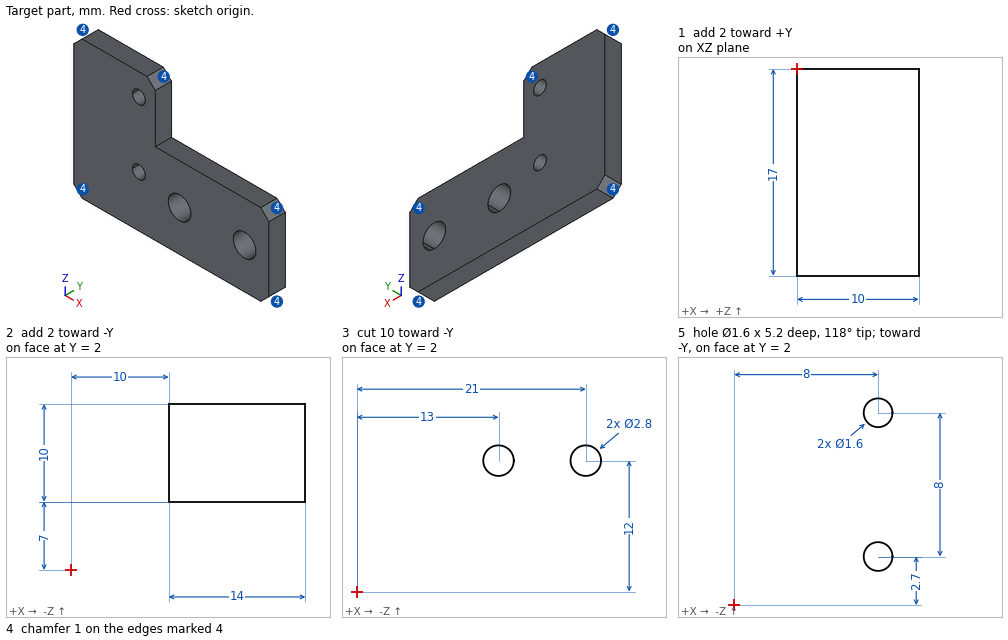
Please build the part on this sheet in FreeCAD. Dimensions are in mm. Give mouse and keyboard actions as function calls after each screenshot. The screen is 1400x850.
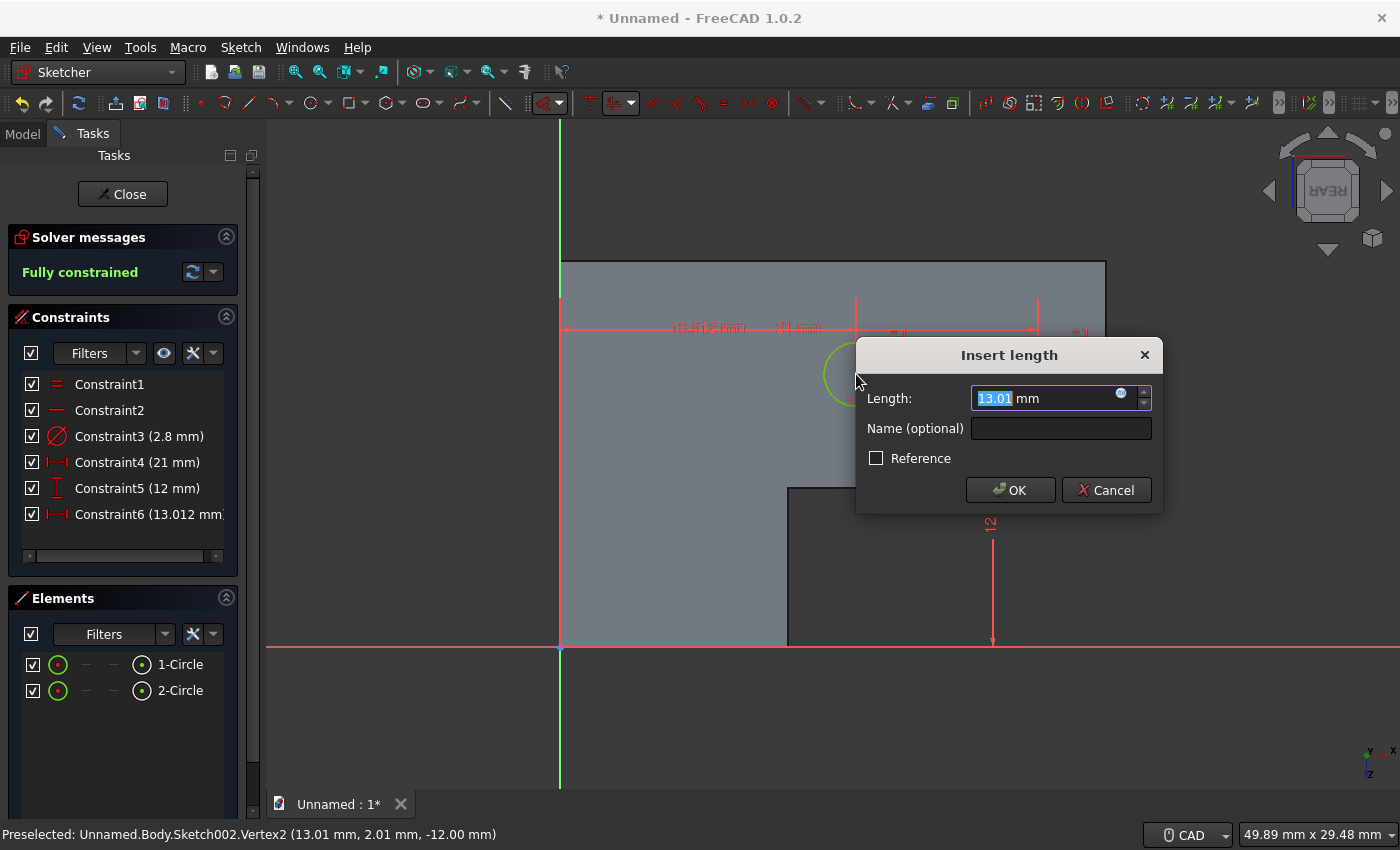
text(13)
key(Return)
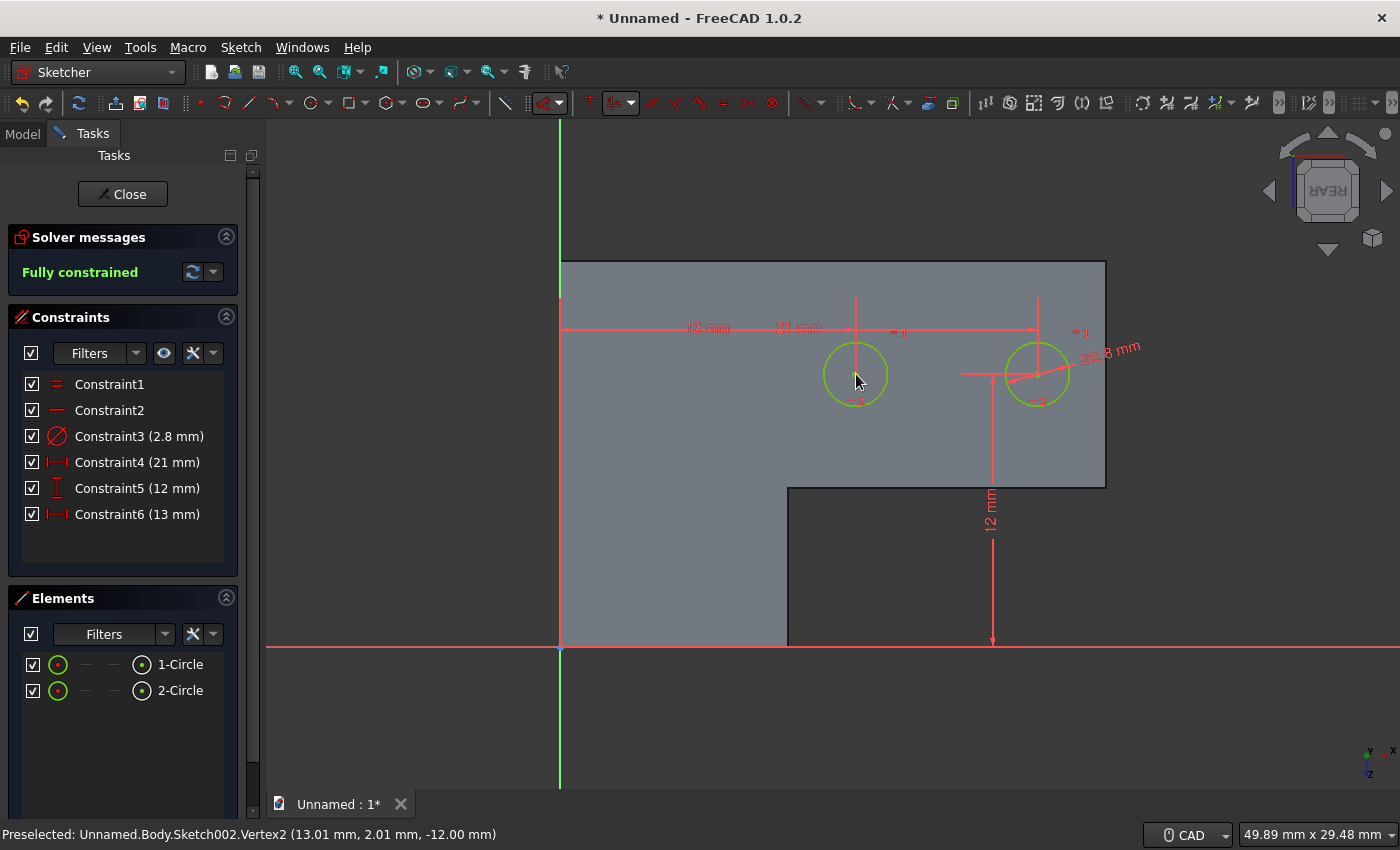
click(123, 194)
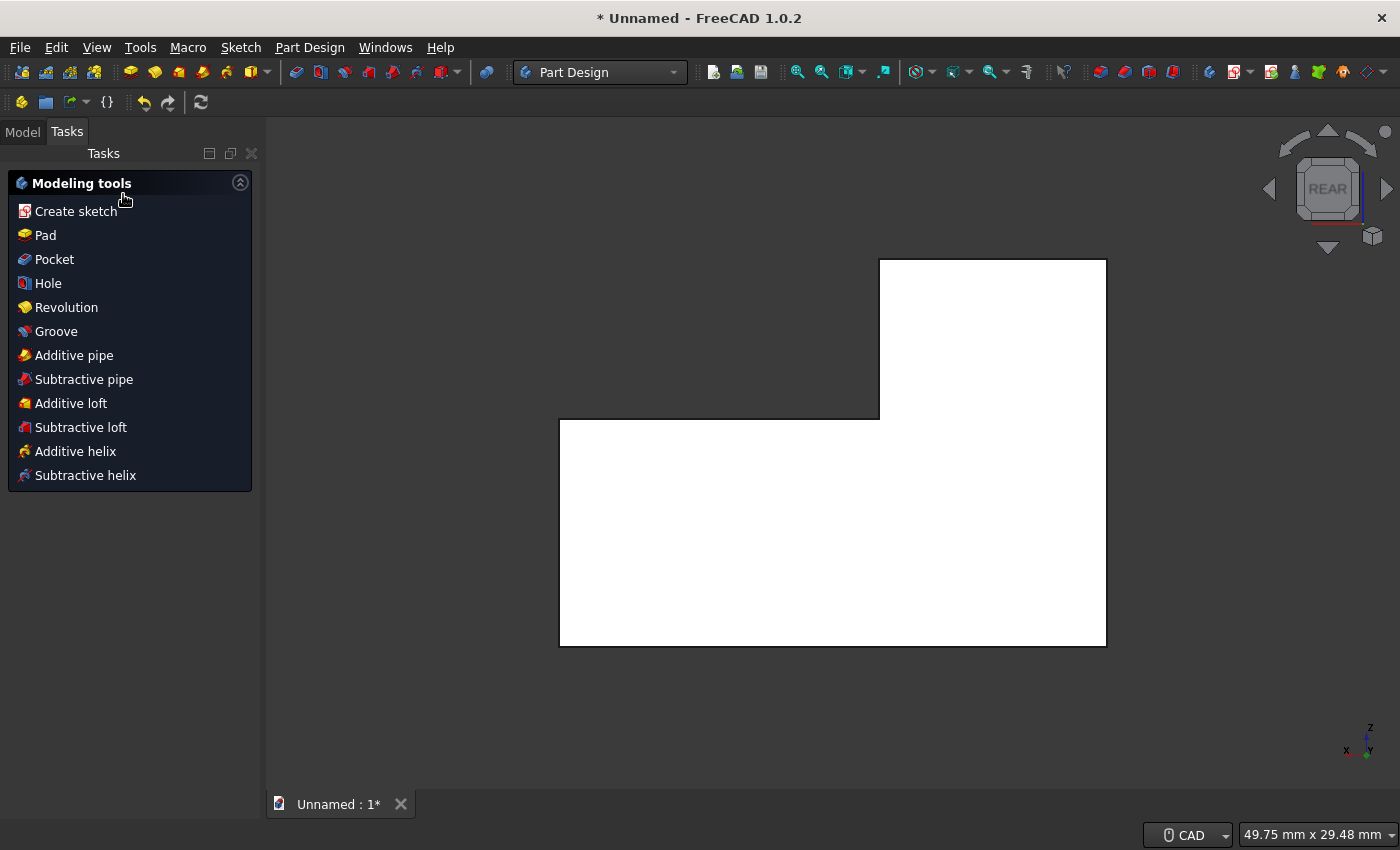
click(298, 72)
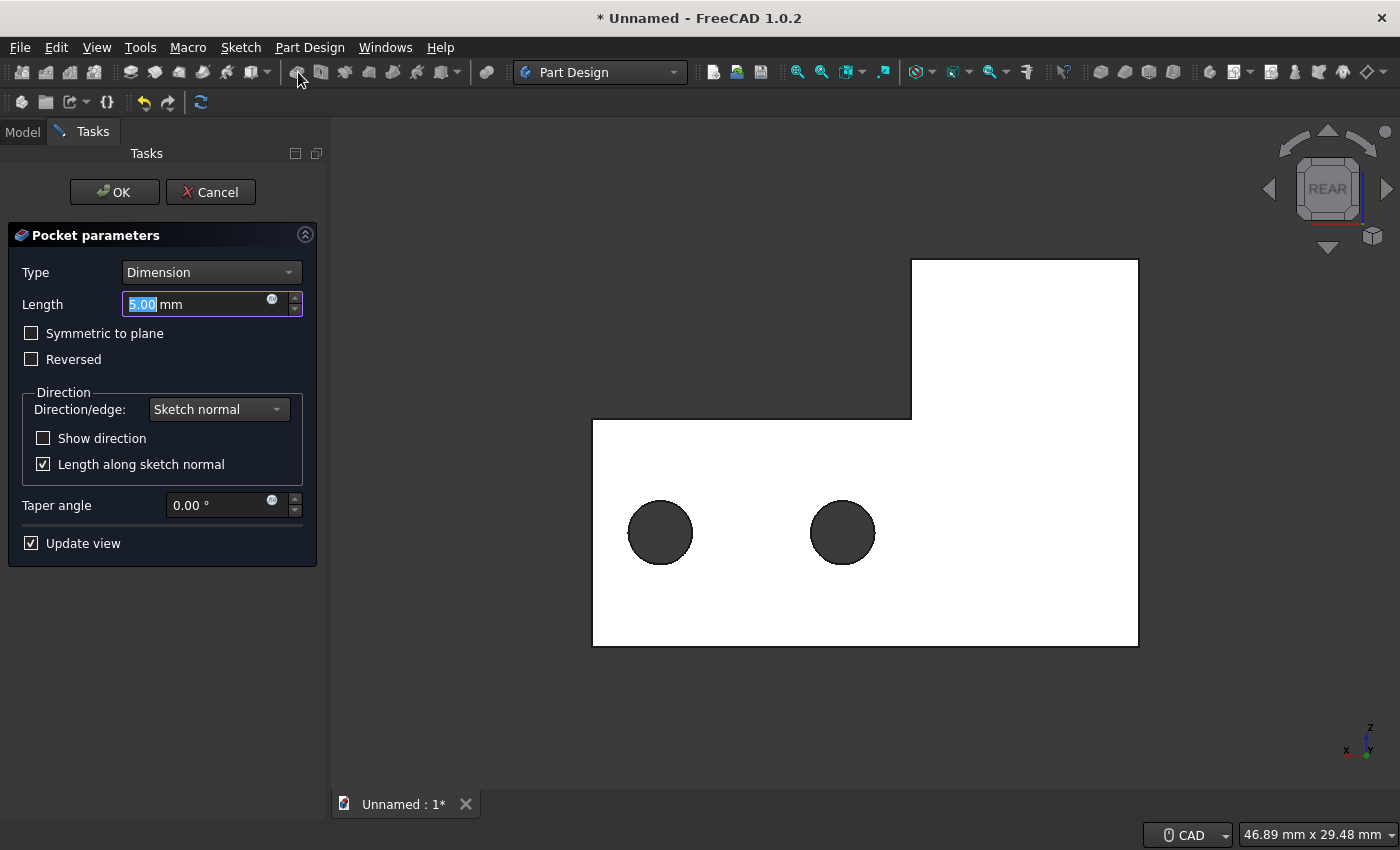
text(10)
key(Tab)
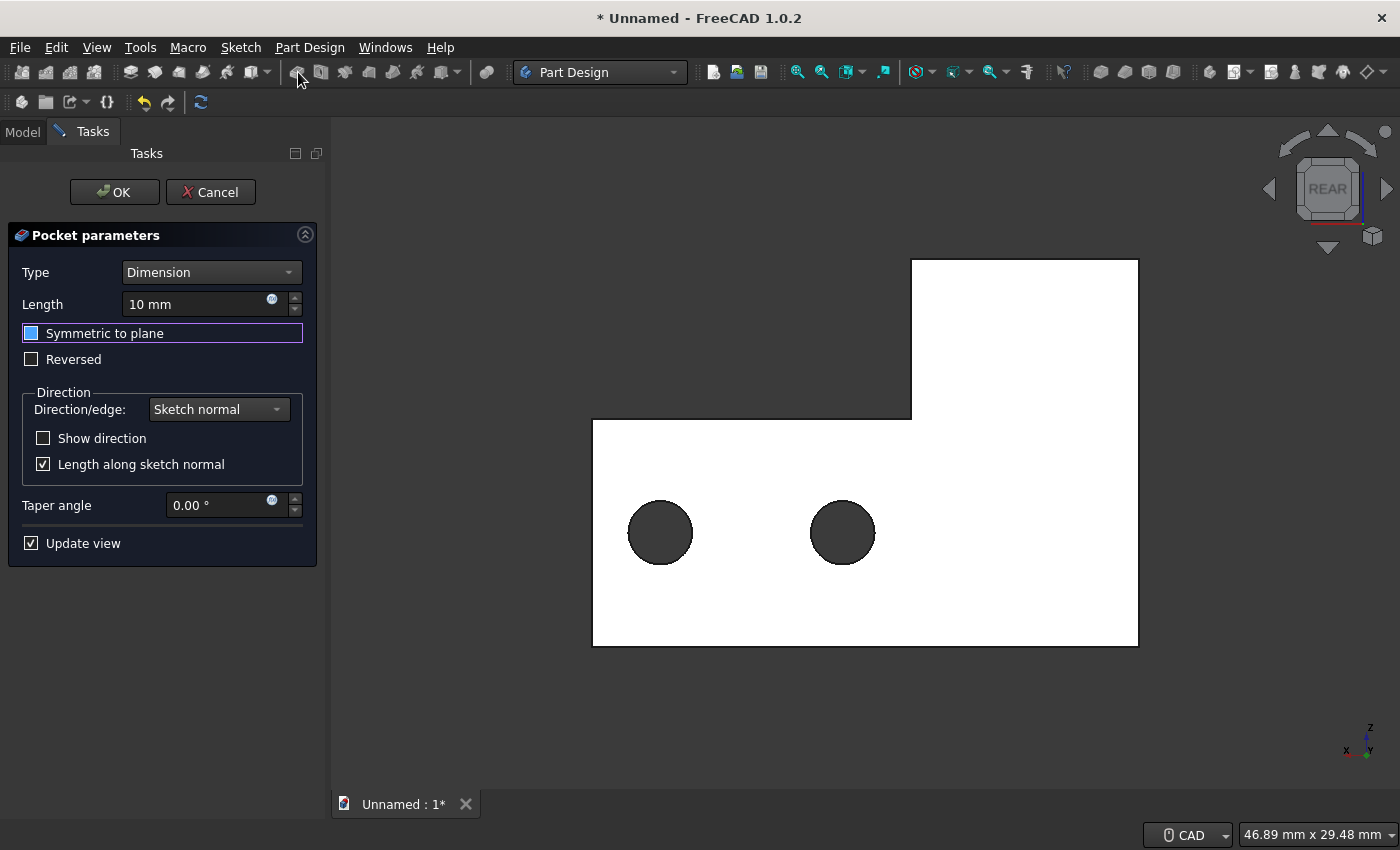
click(115, 192)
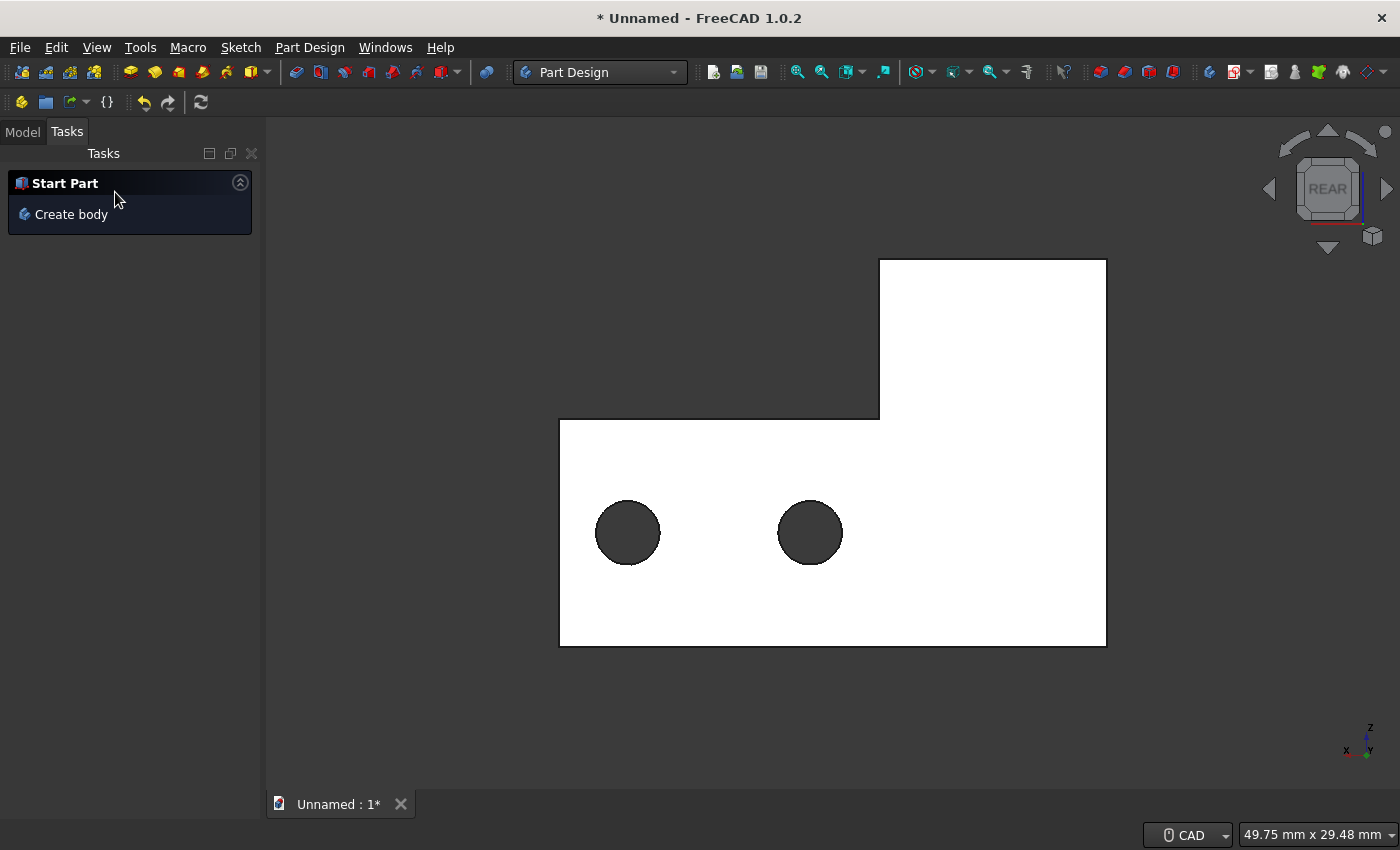
key(0)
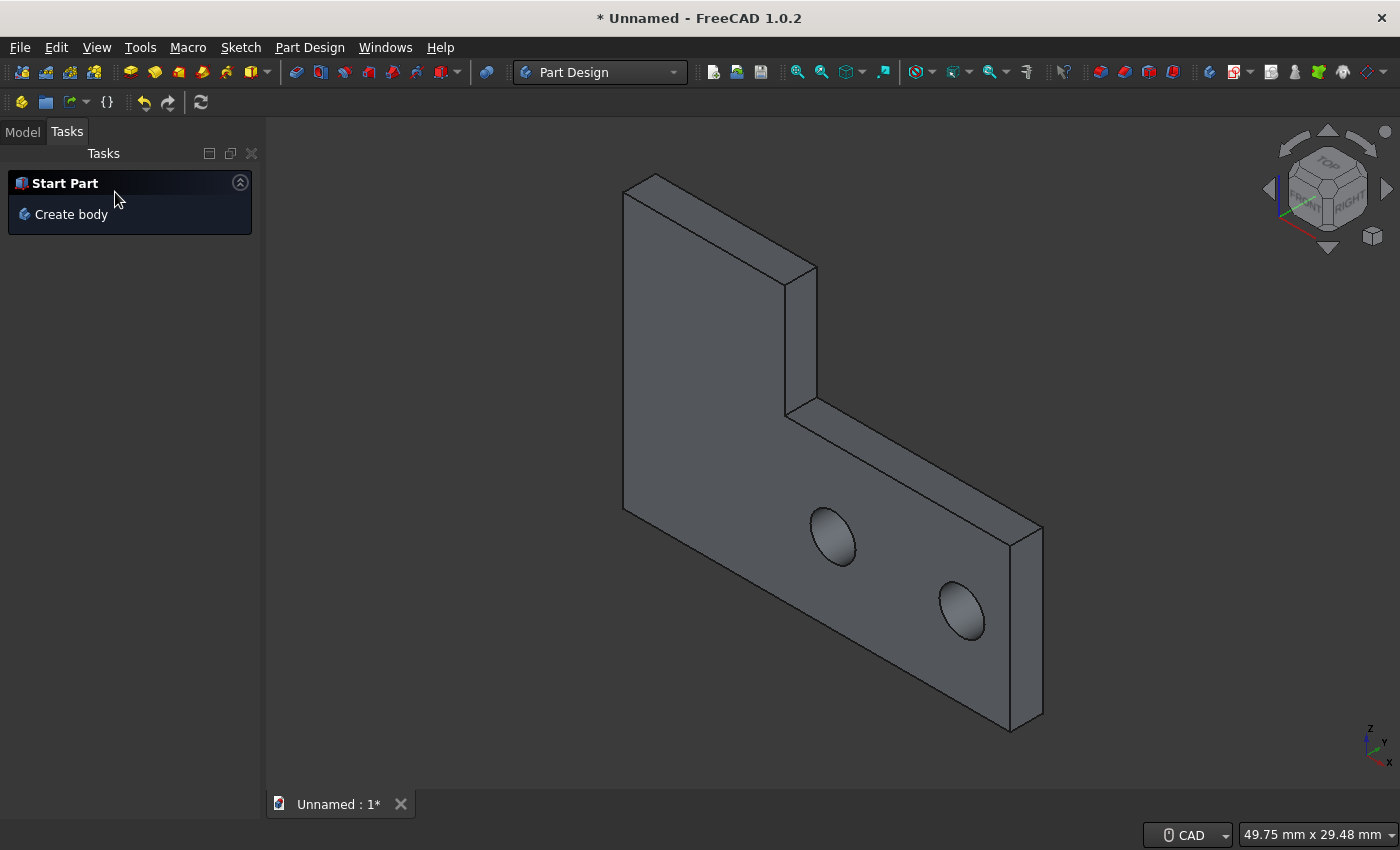
click(801, 275)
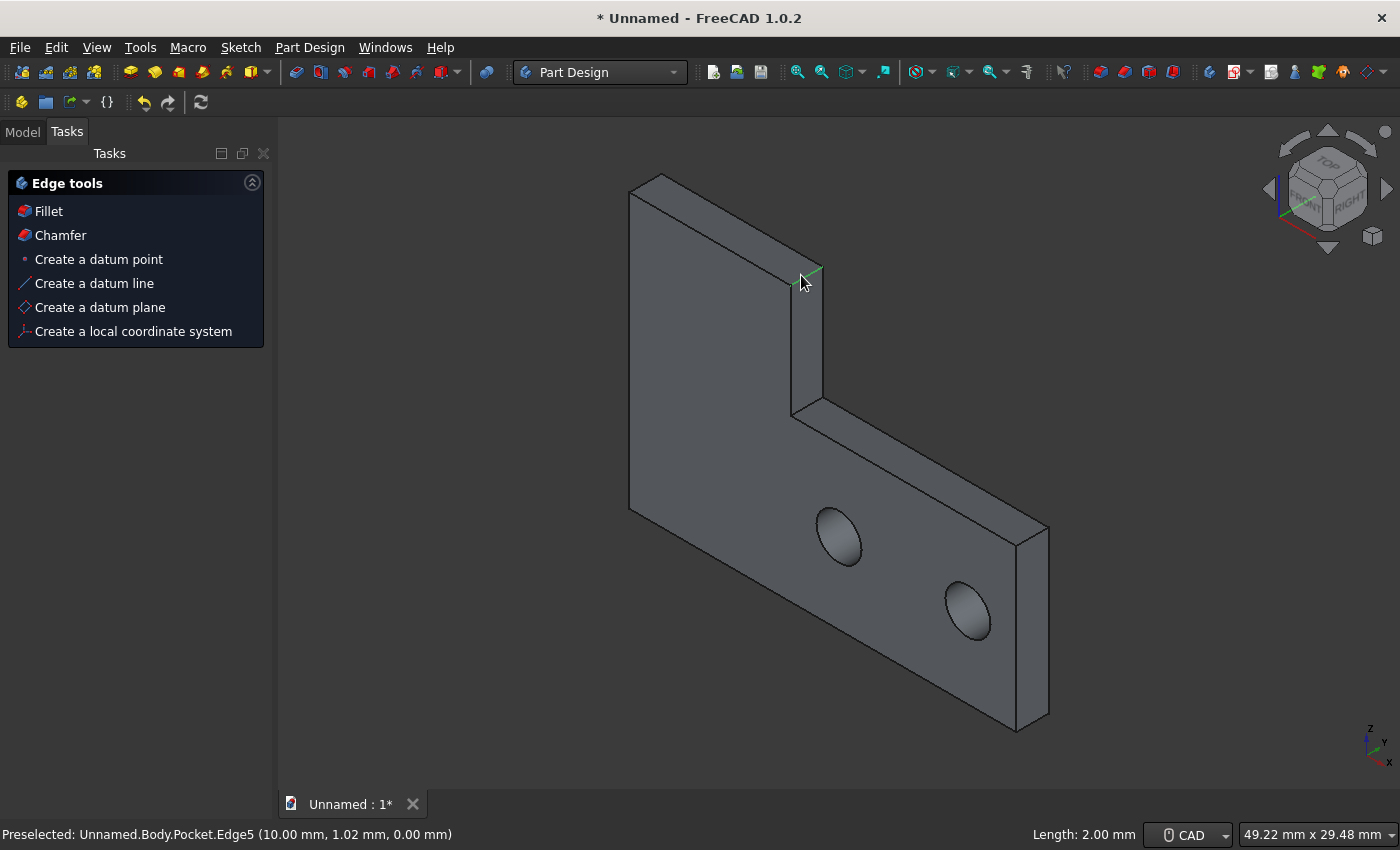
click(1032, 536, ctrl)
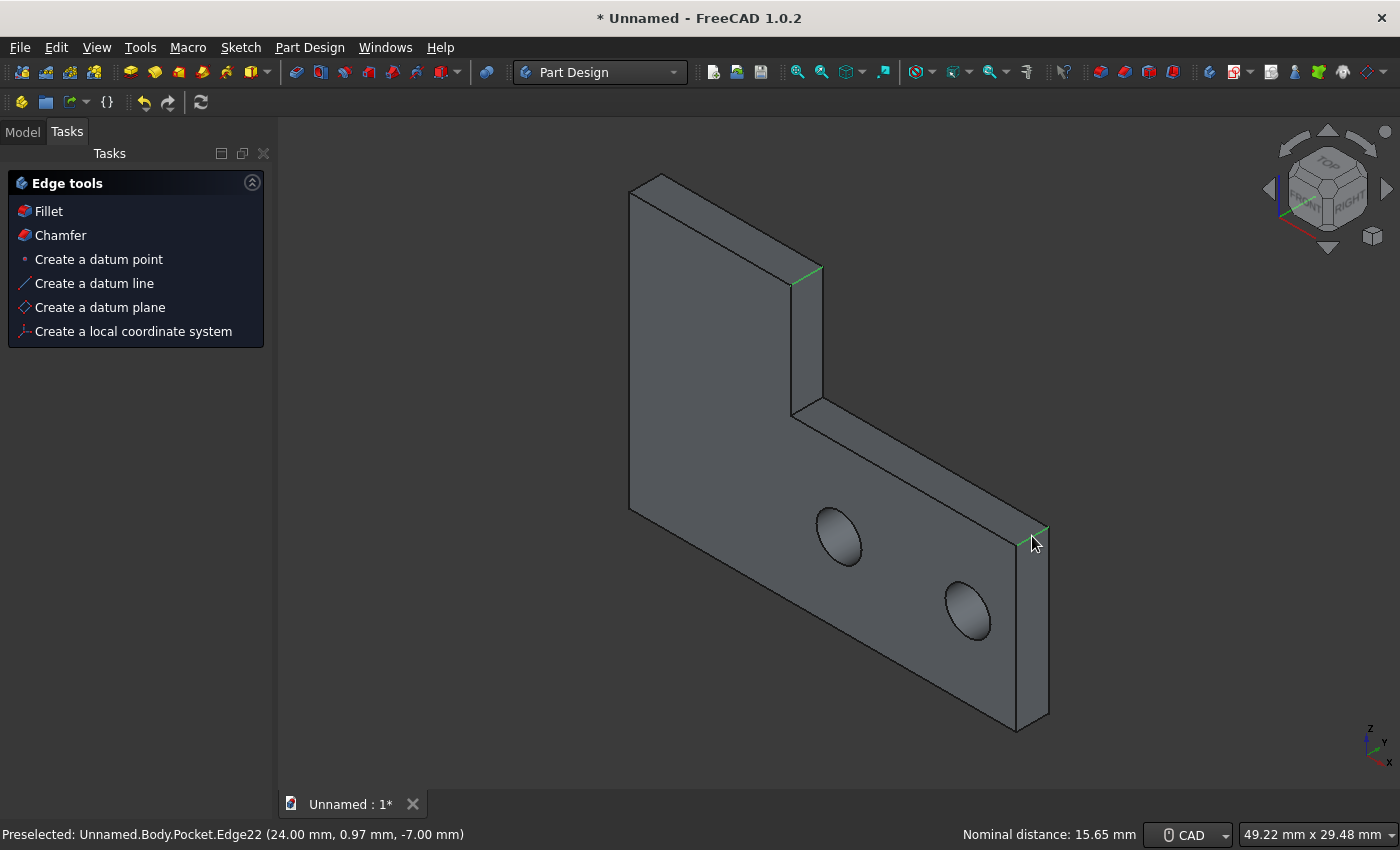
key(2)